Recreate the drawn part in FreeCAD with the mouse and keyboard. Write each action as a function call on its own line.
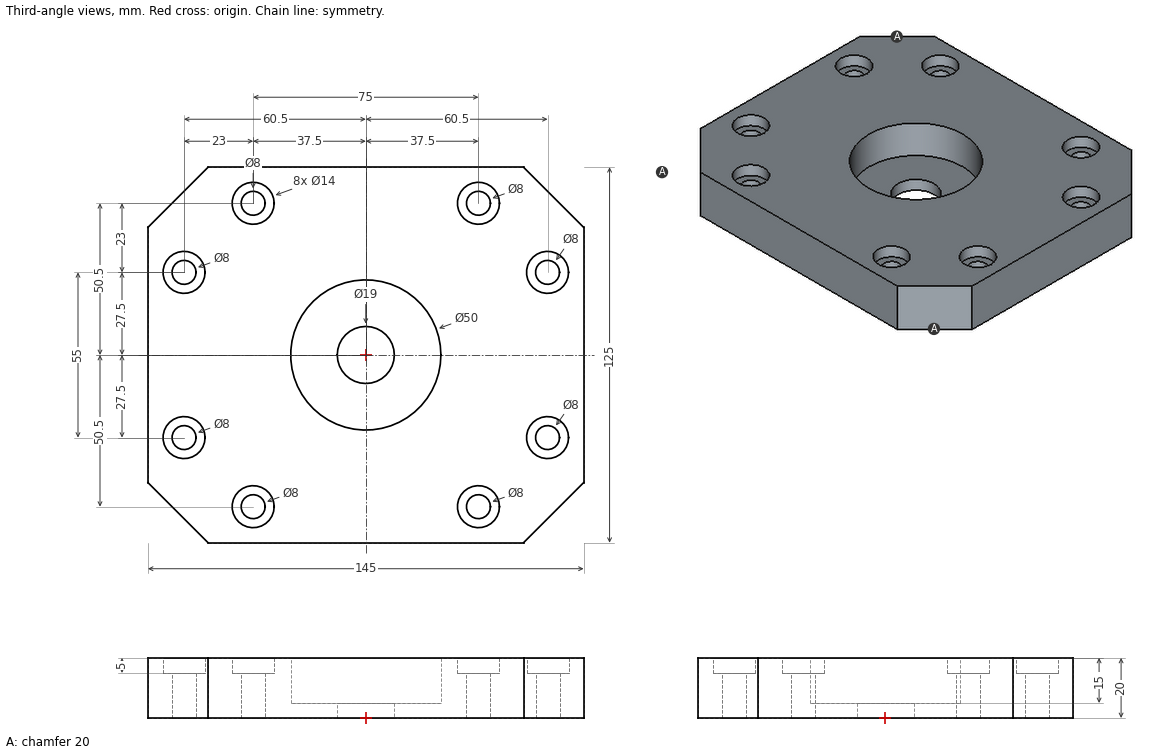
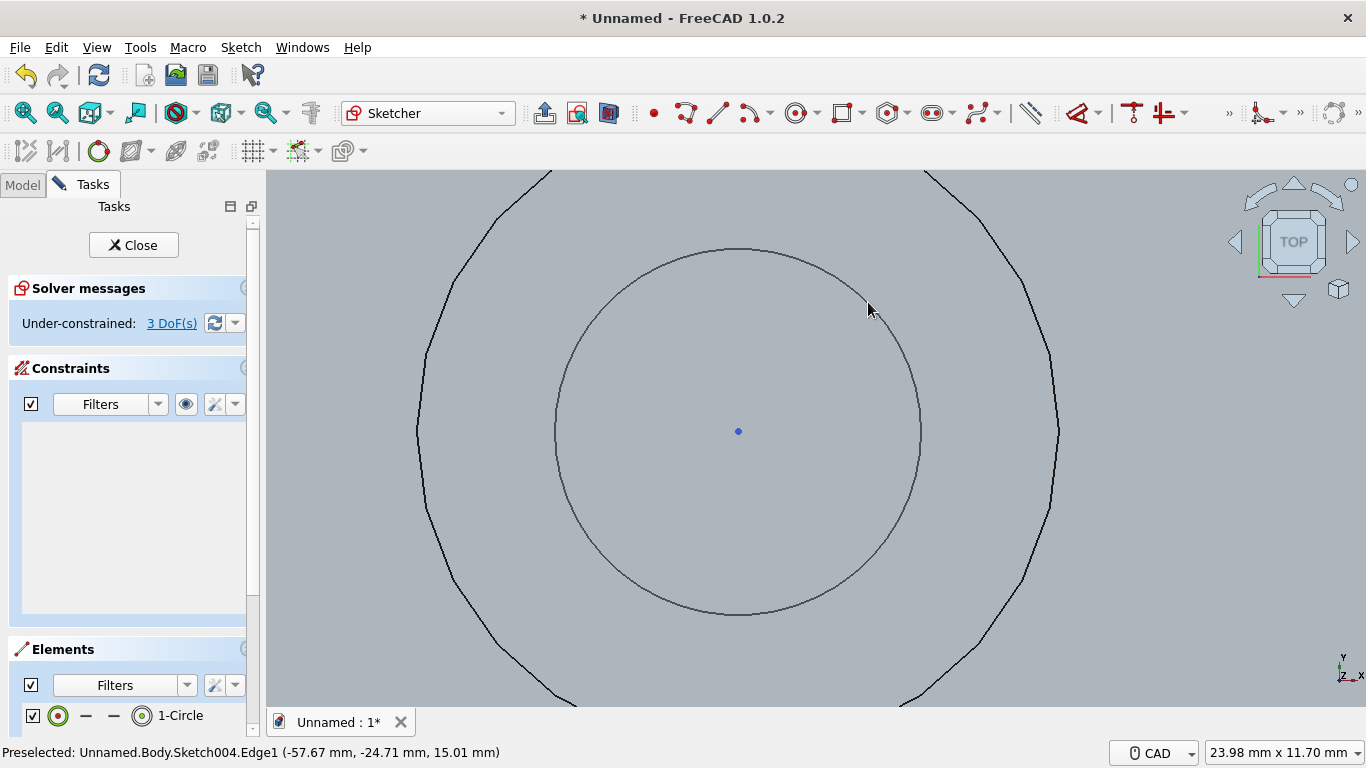
click(1078, 114)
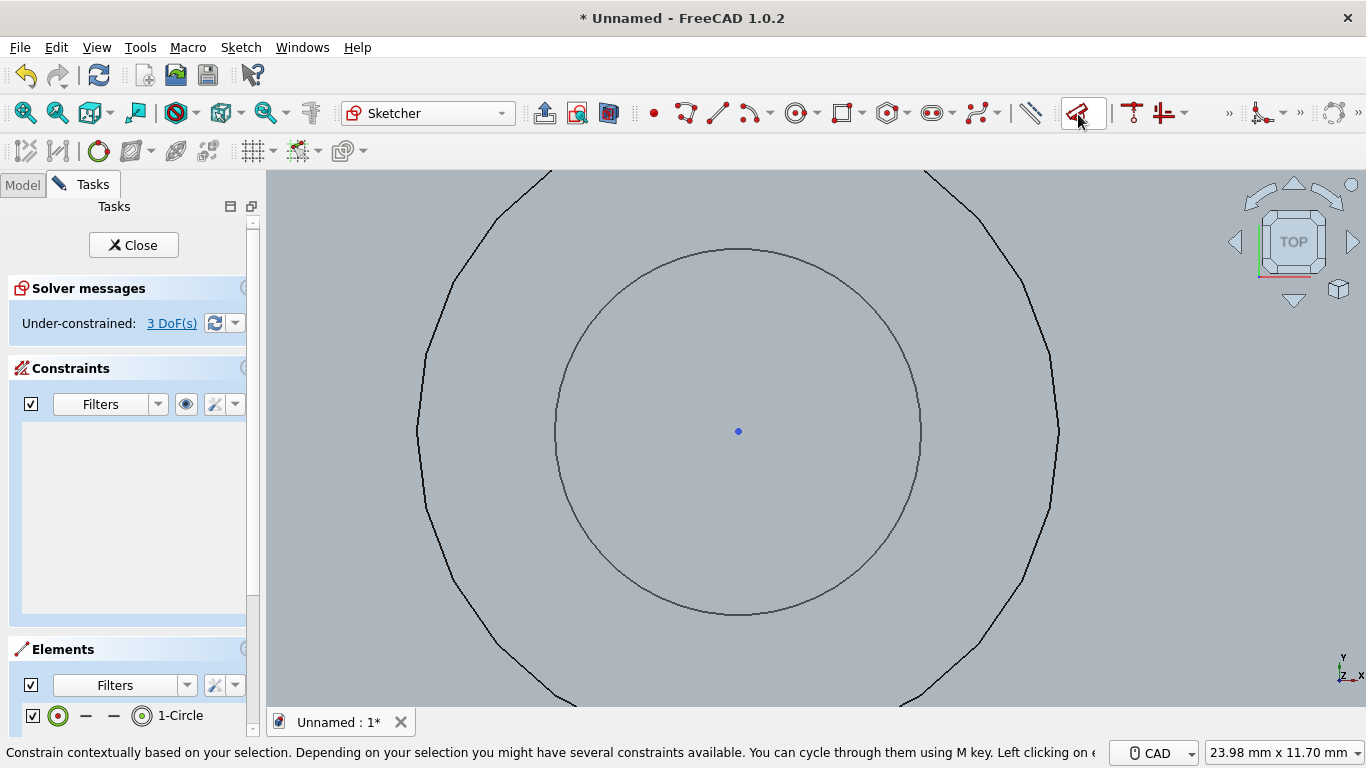
click(867, 302)
click(890, 279)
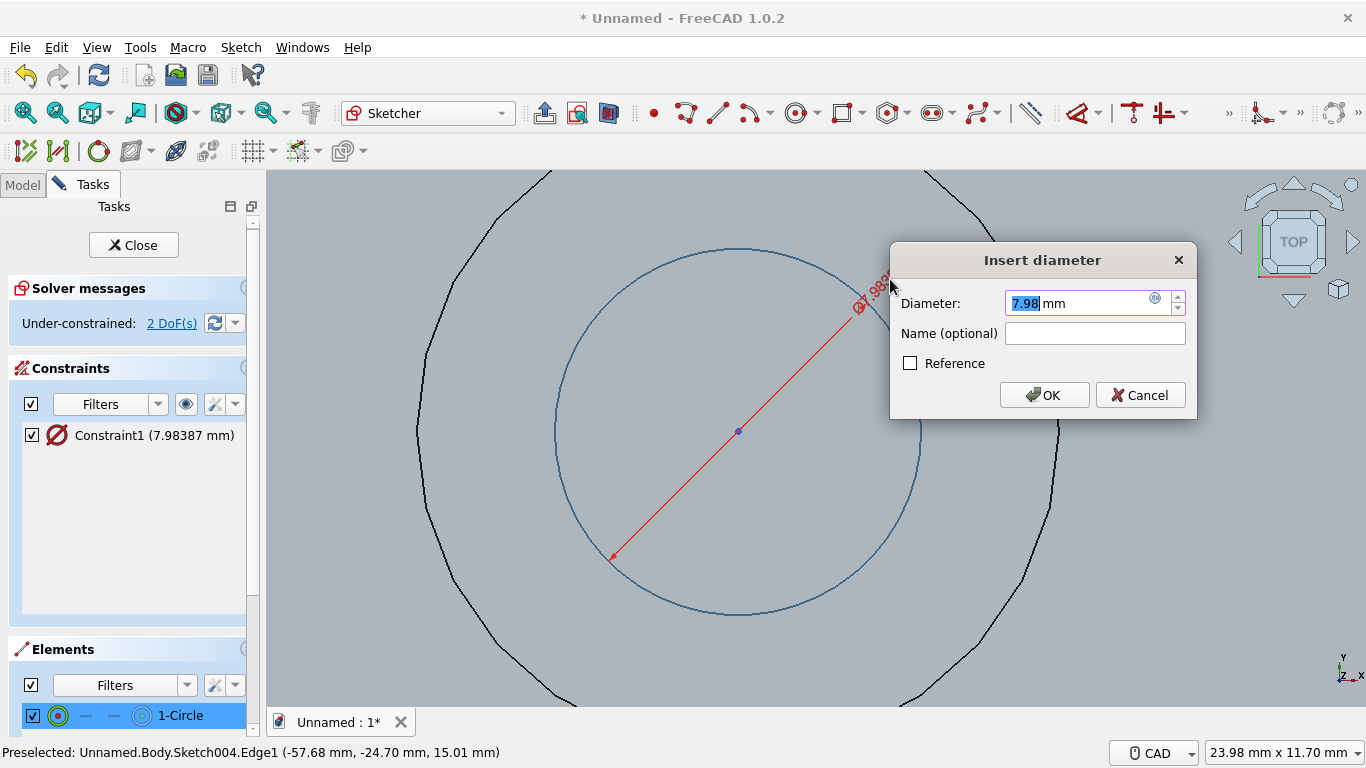
text(8)
key(Return)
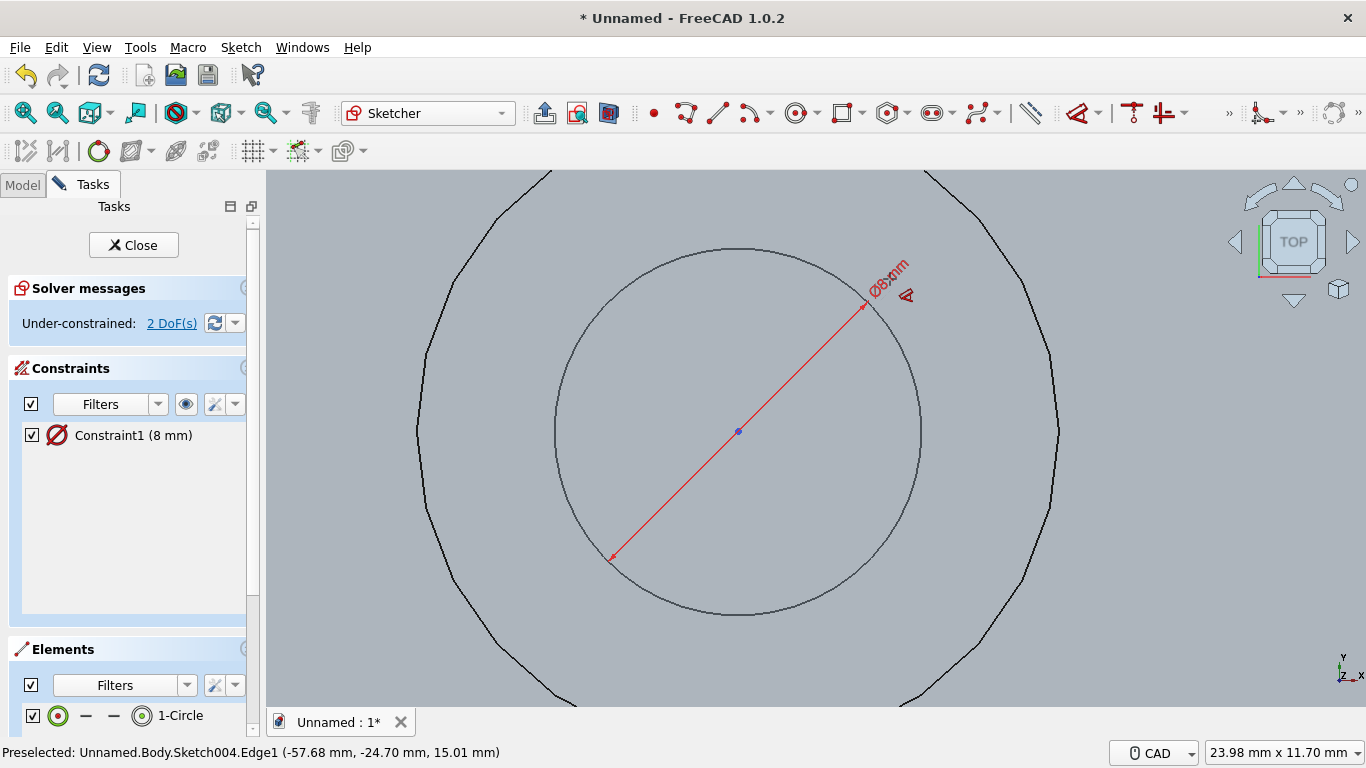
click(738, 432)
click(970, 466)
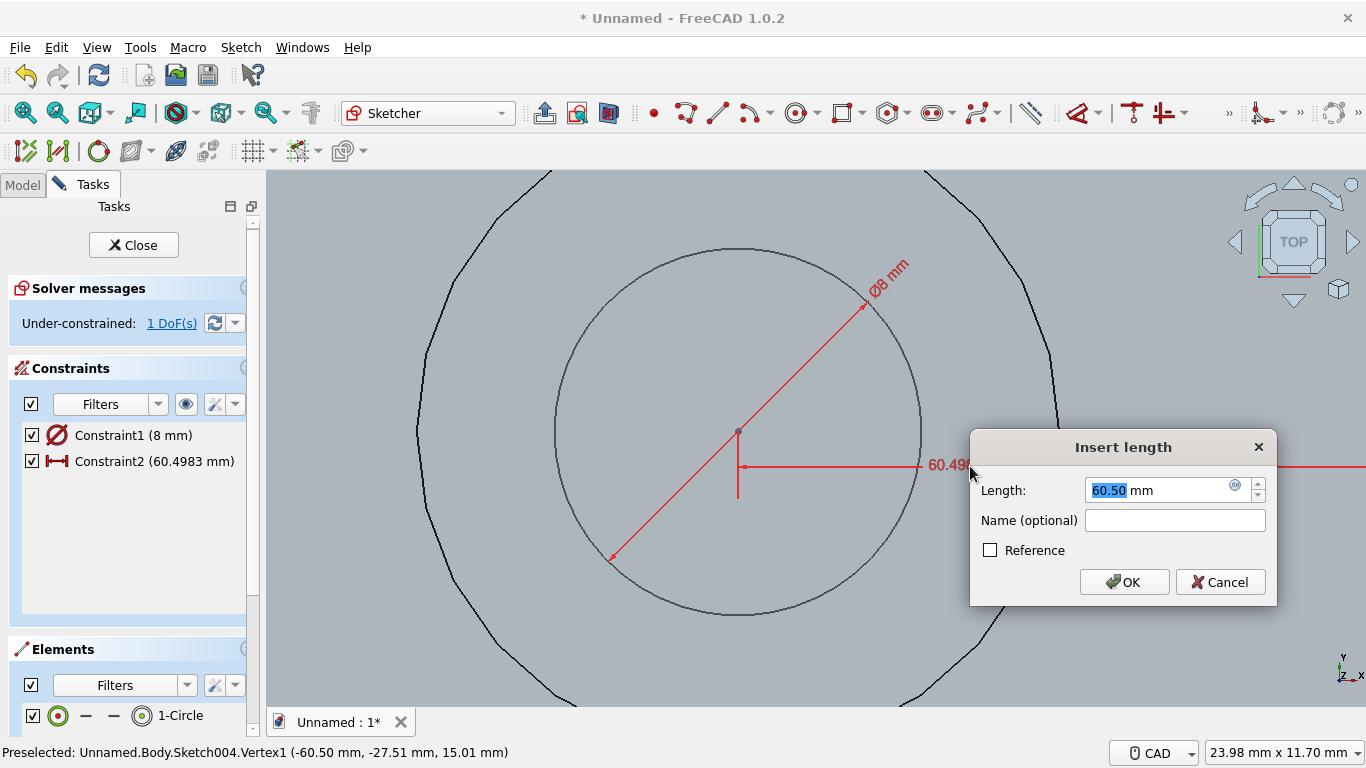
text(60.5)
key(Return)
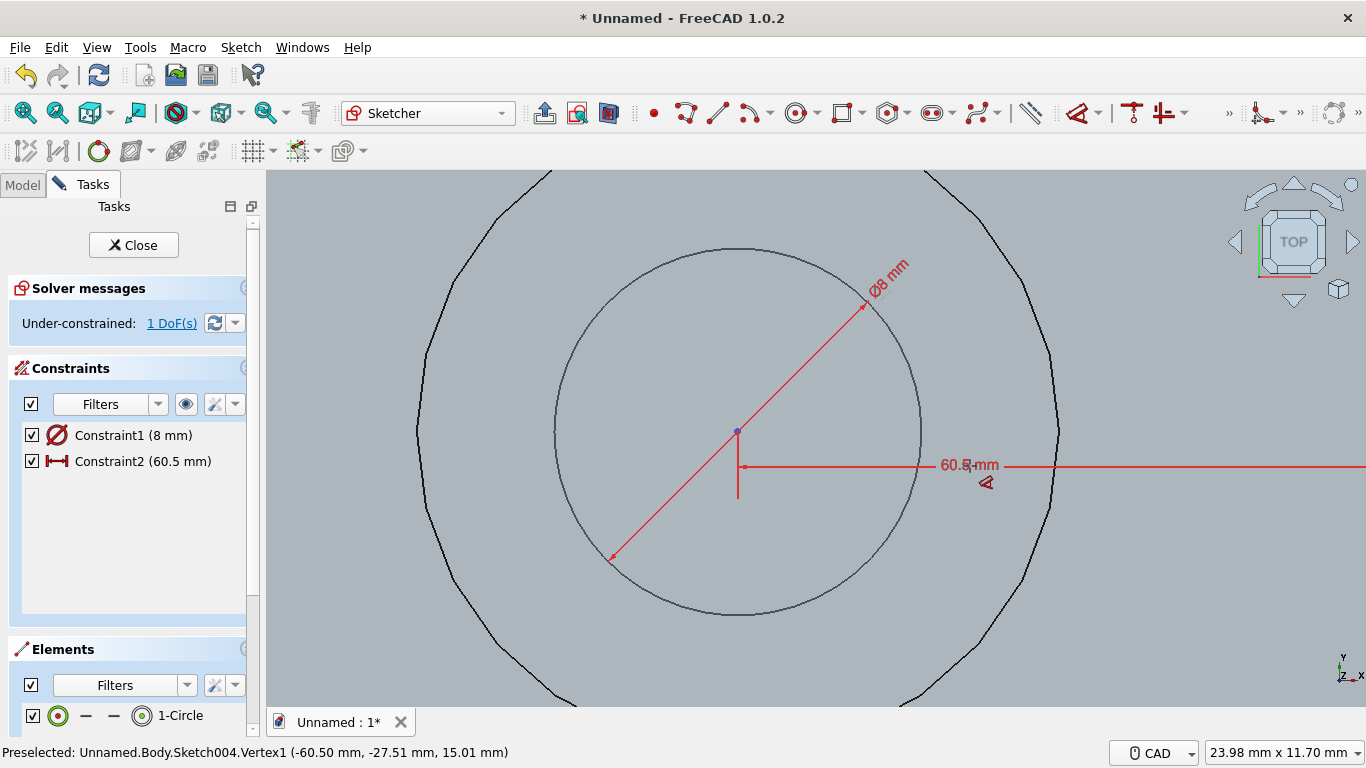
click(738, 432)
click(704, 315)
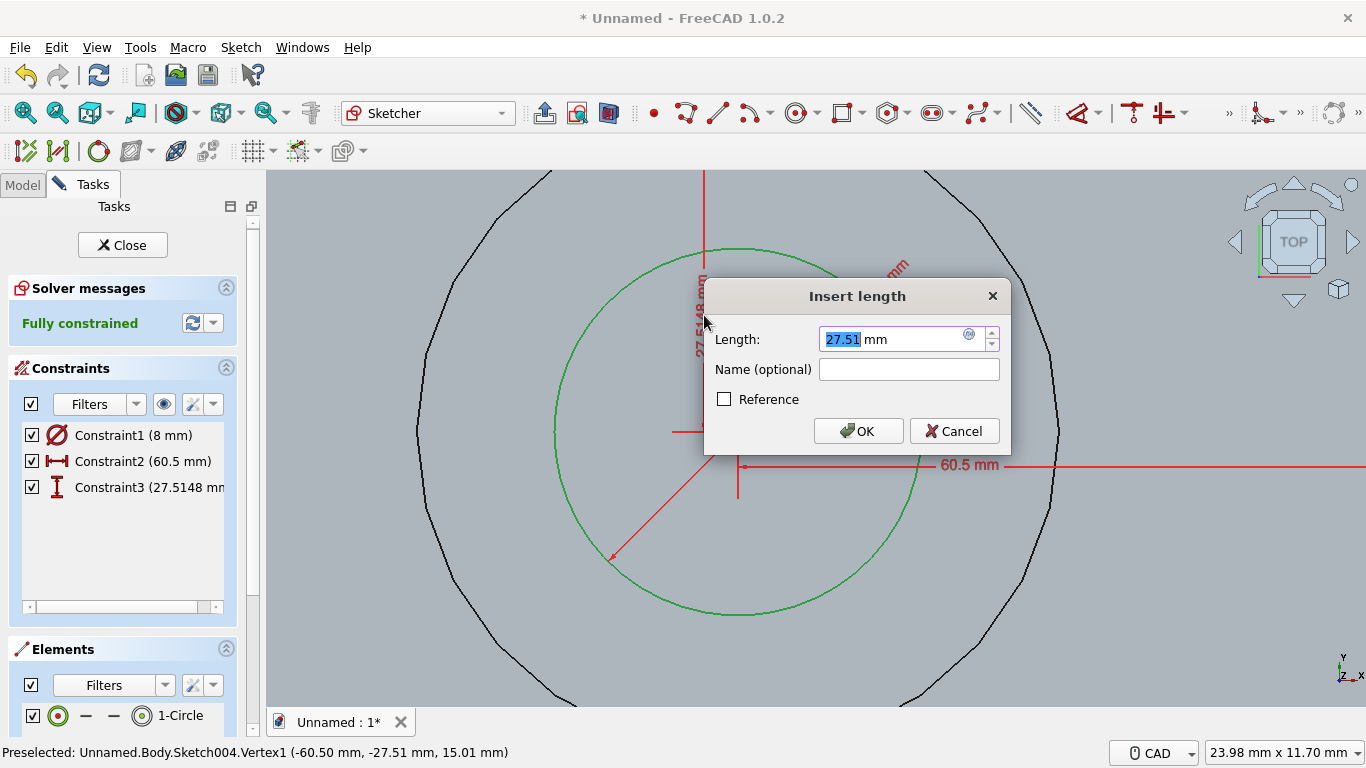
text(27.5)
key(Return)
key(Escape)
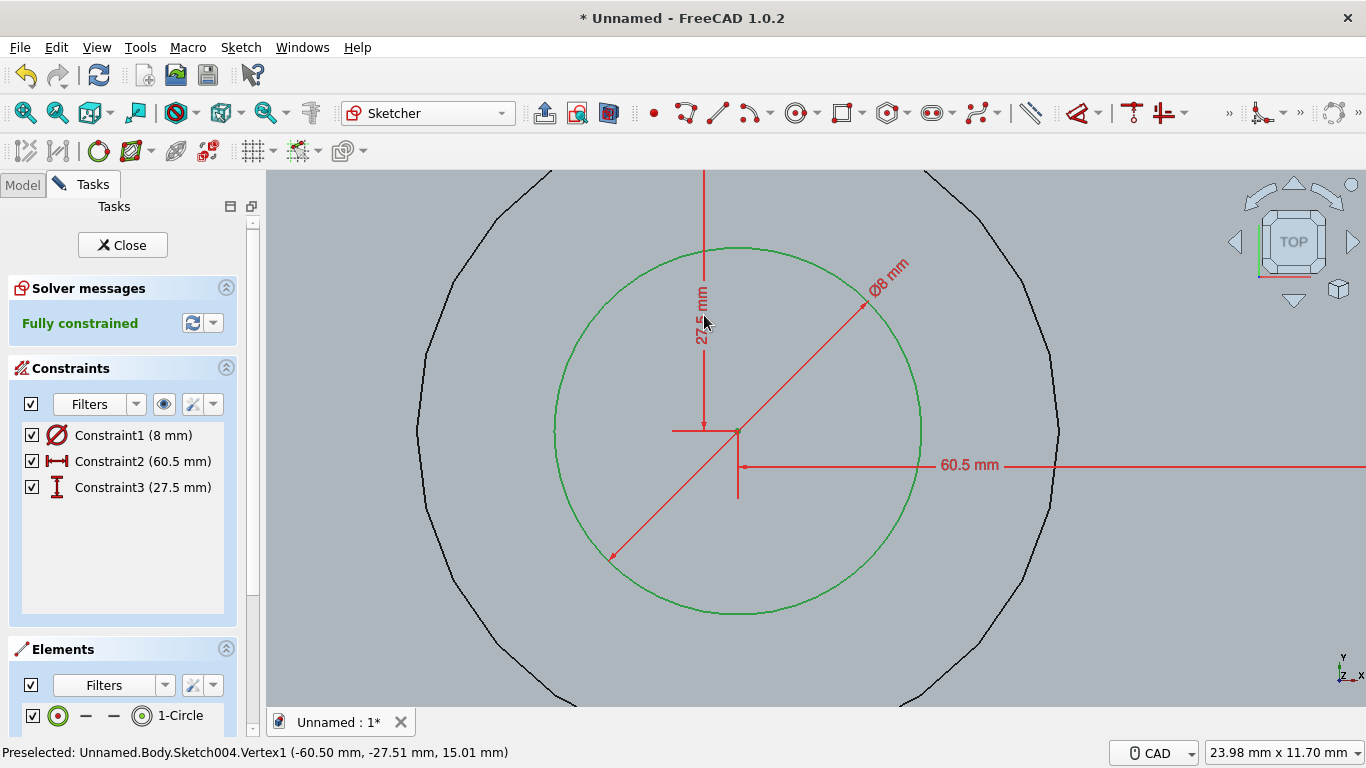
click(123, 245)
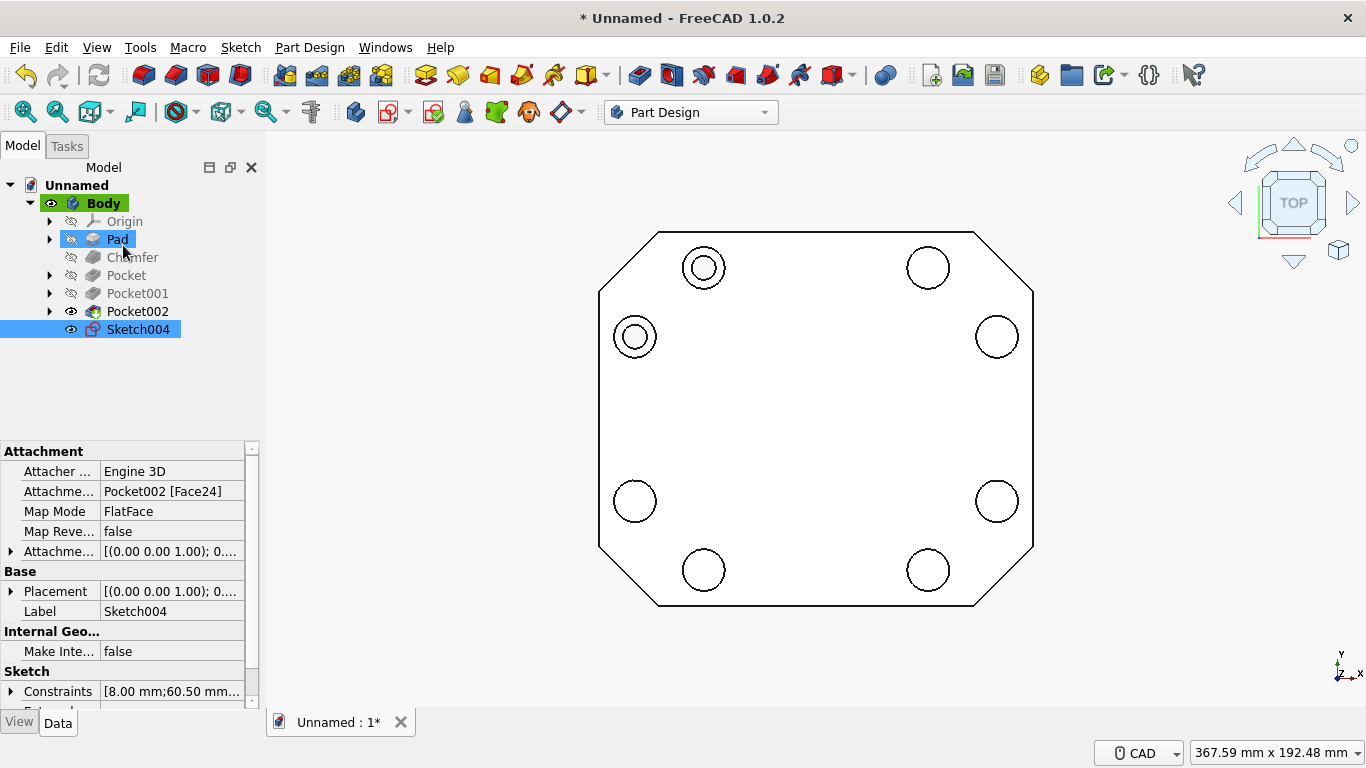
click(640, 76)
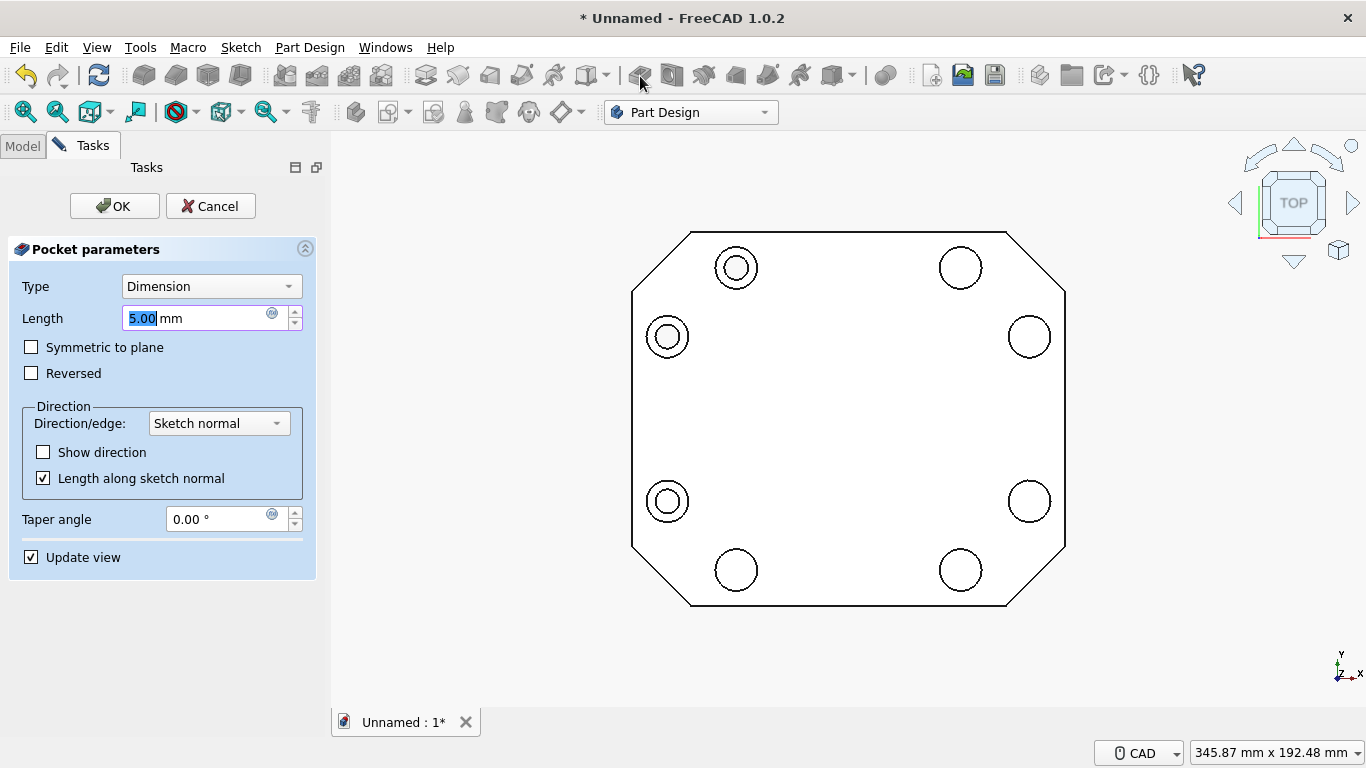
click(212, 286)